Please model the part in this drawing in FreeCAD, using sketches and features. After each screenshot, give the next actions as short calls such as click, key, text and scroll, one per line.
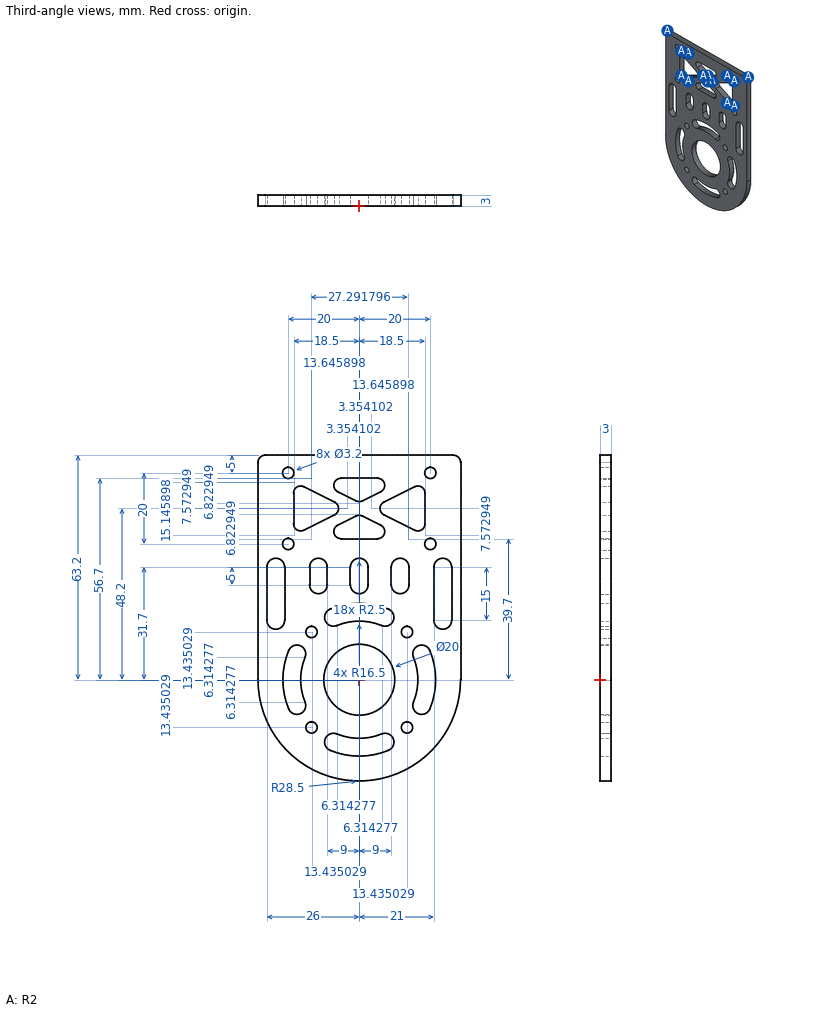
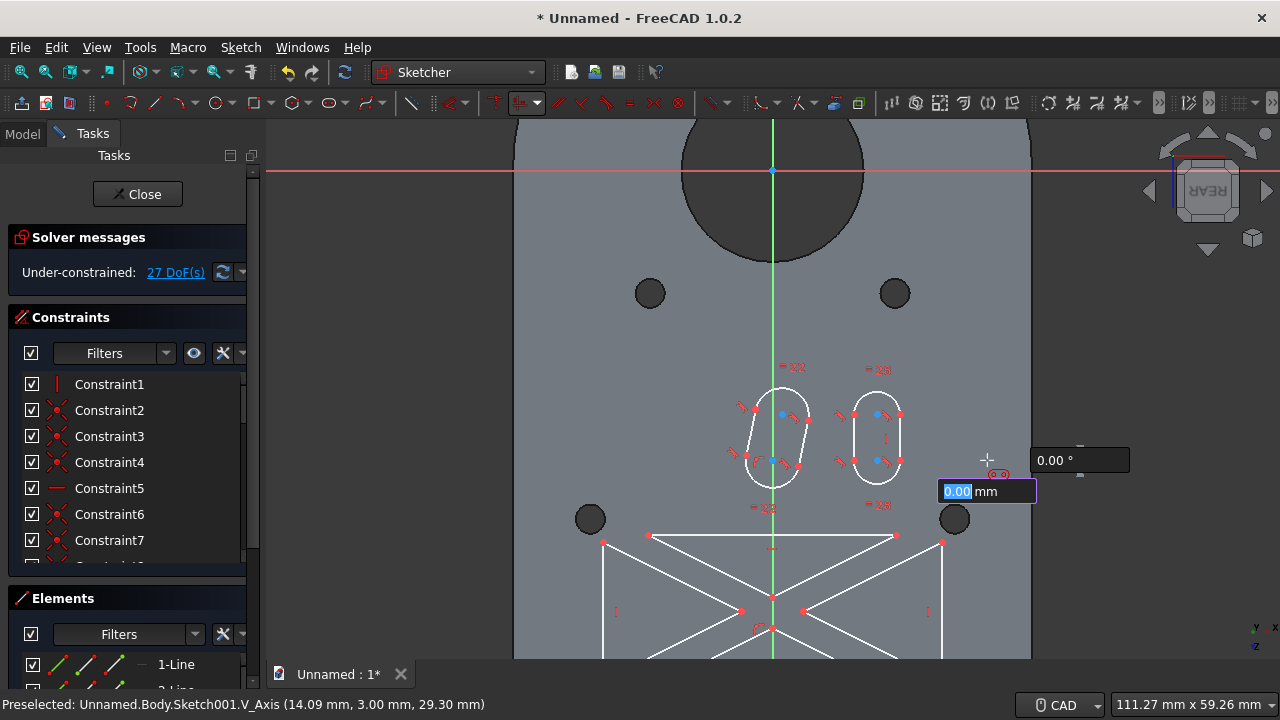
click(987, 323)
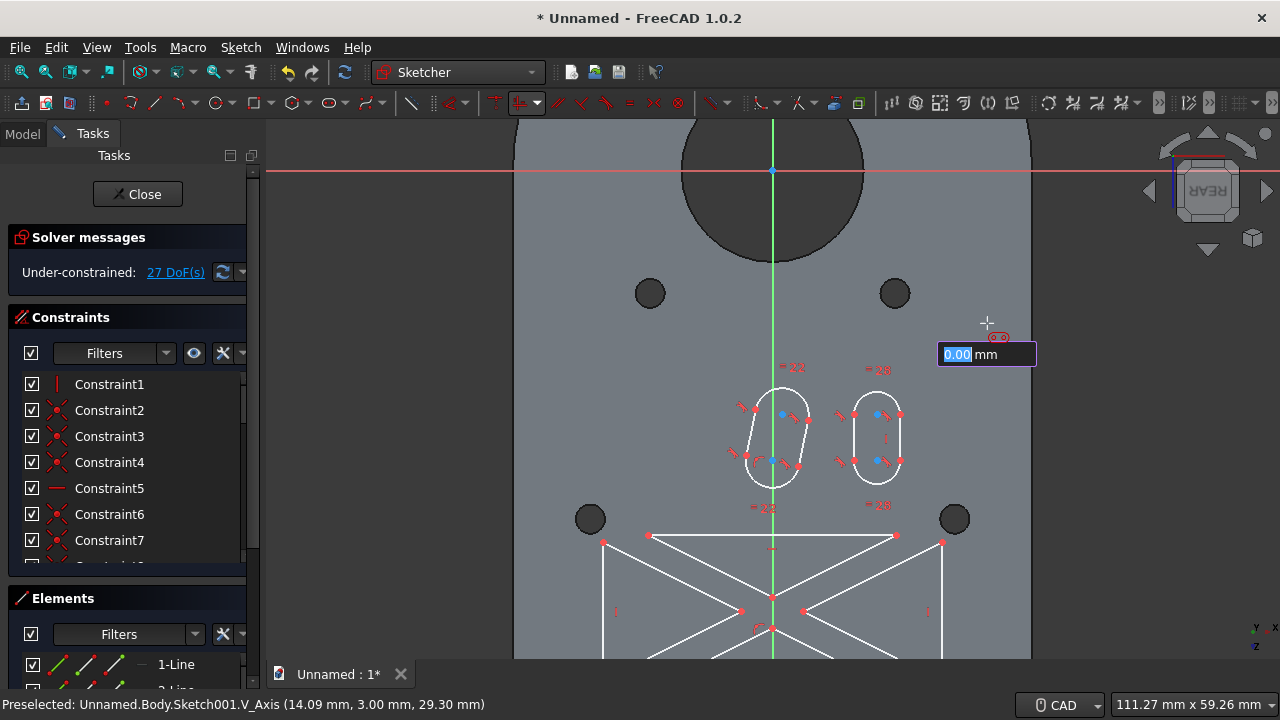
click(1010, 391)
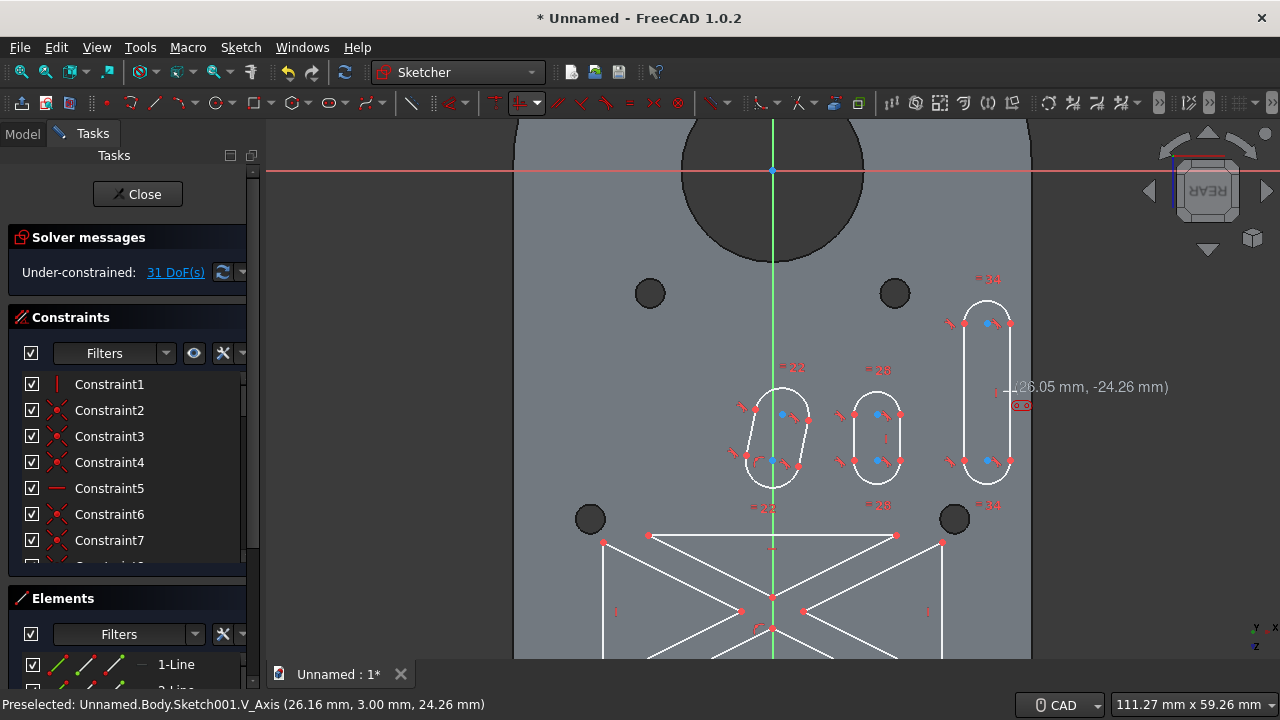
click(180, 104)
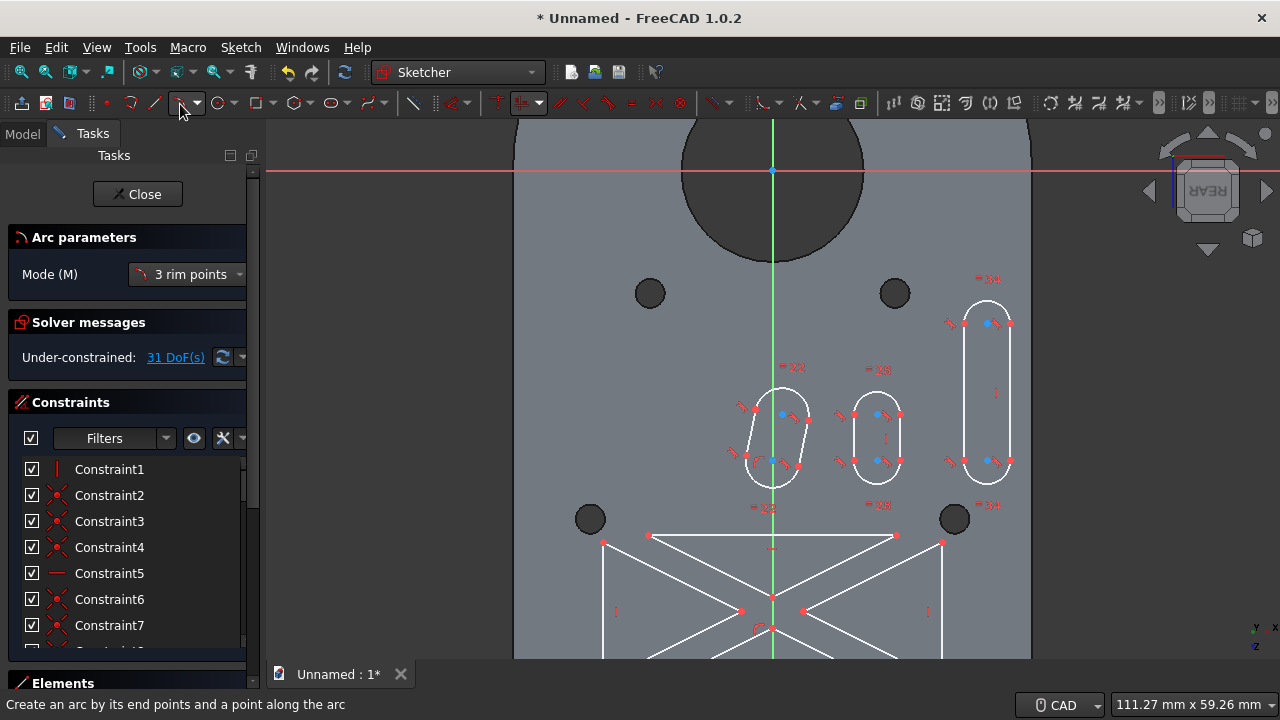
click(830, 310)
click(715, 310)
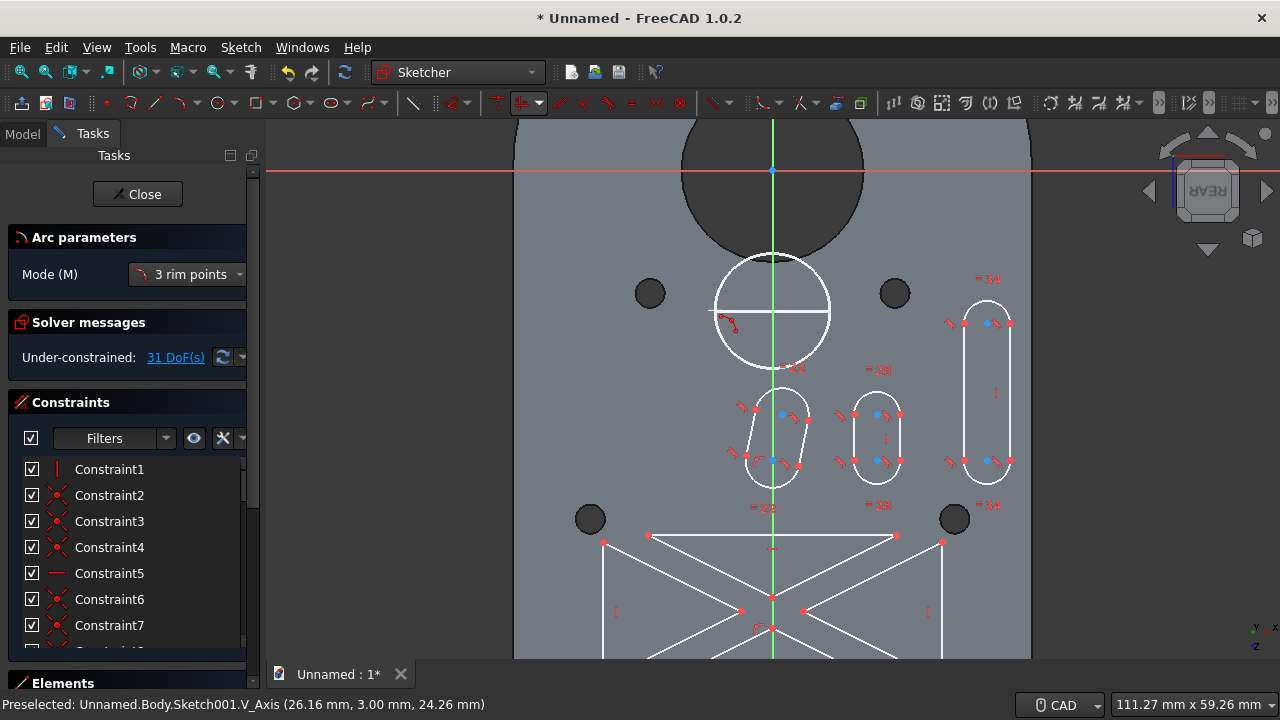
scroll(761, 321, up, 2)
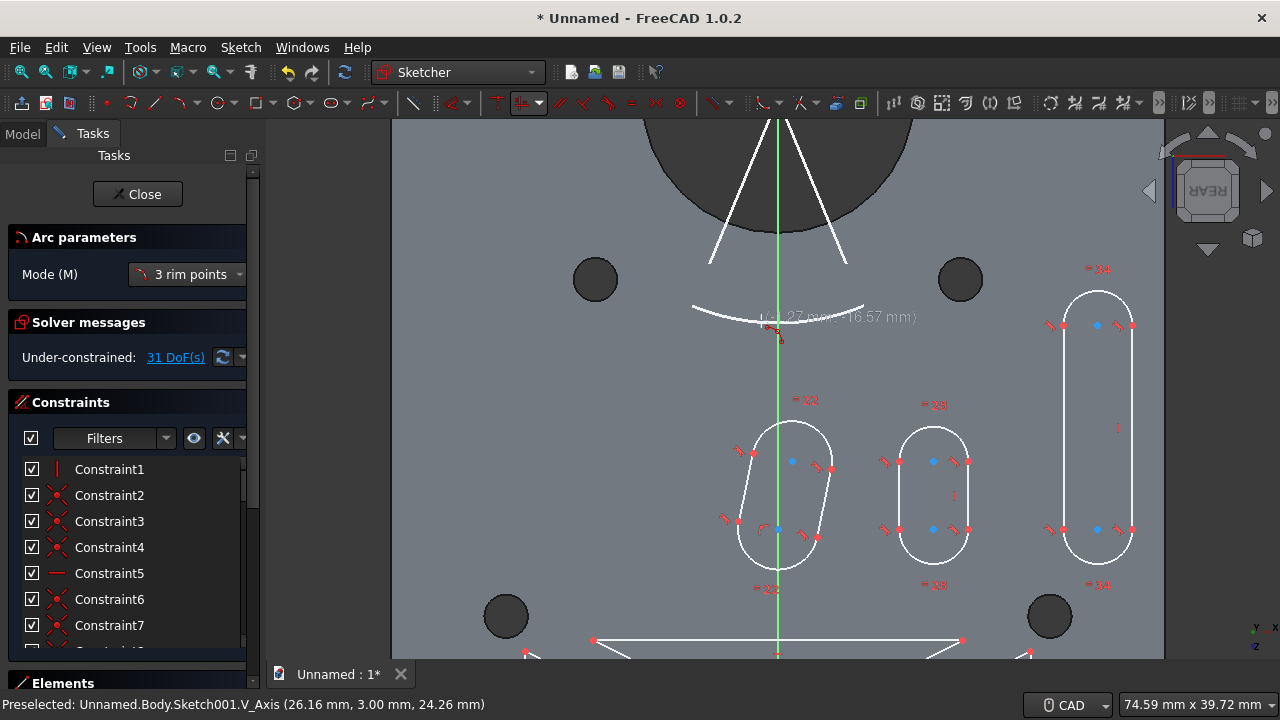
click(760, 321)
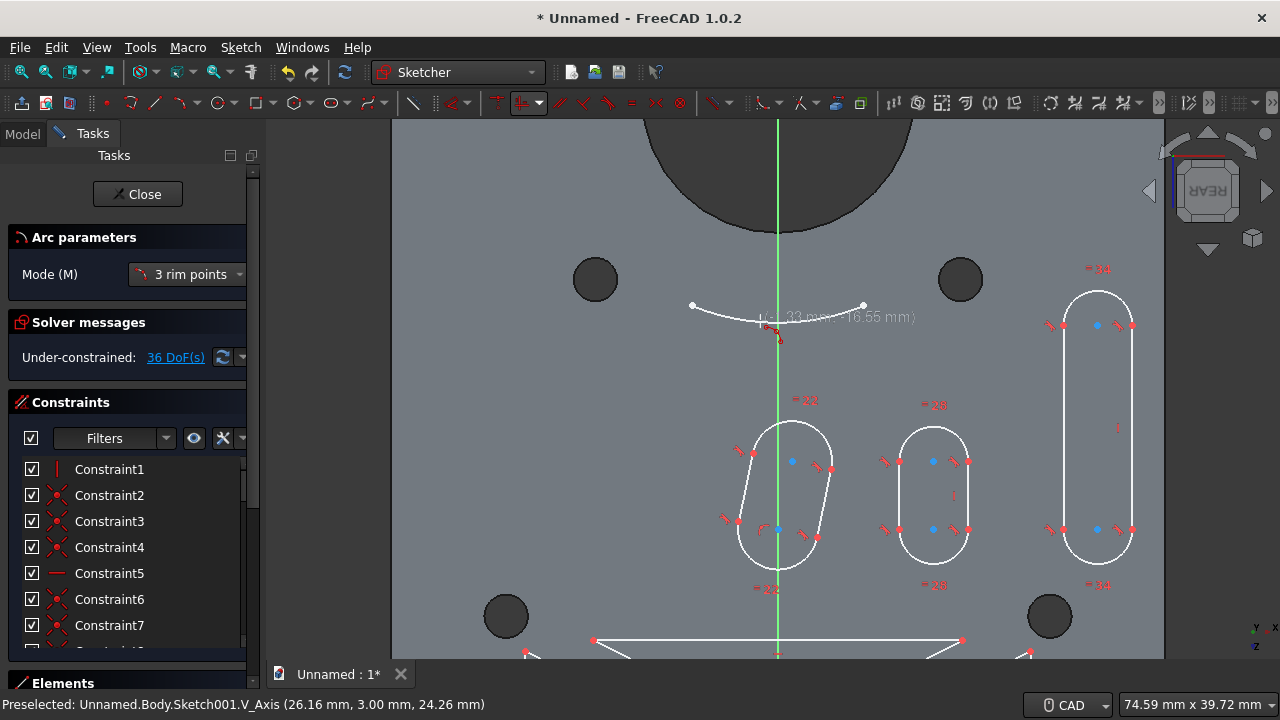
click(692, 306)
click(666, 367)
click(648, 323)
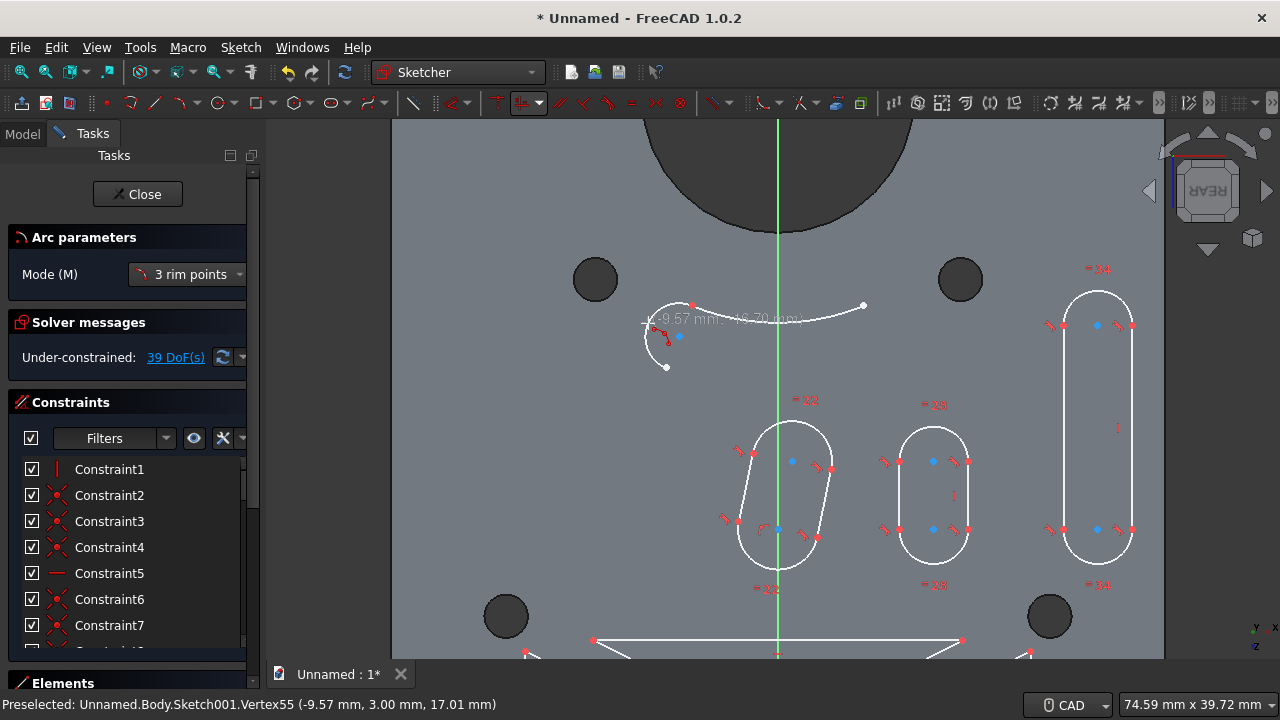
click(666, 368)
click(890, 367)
click(755, 388)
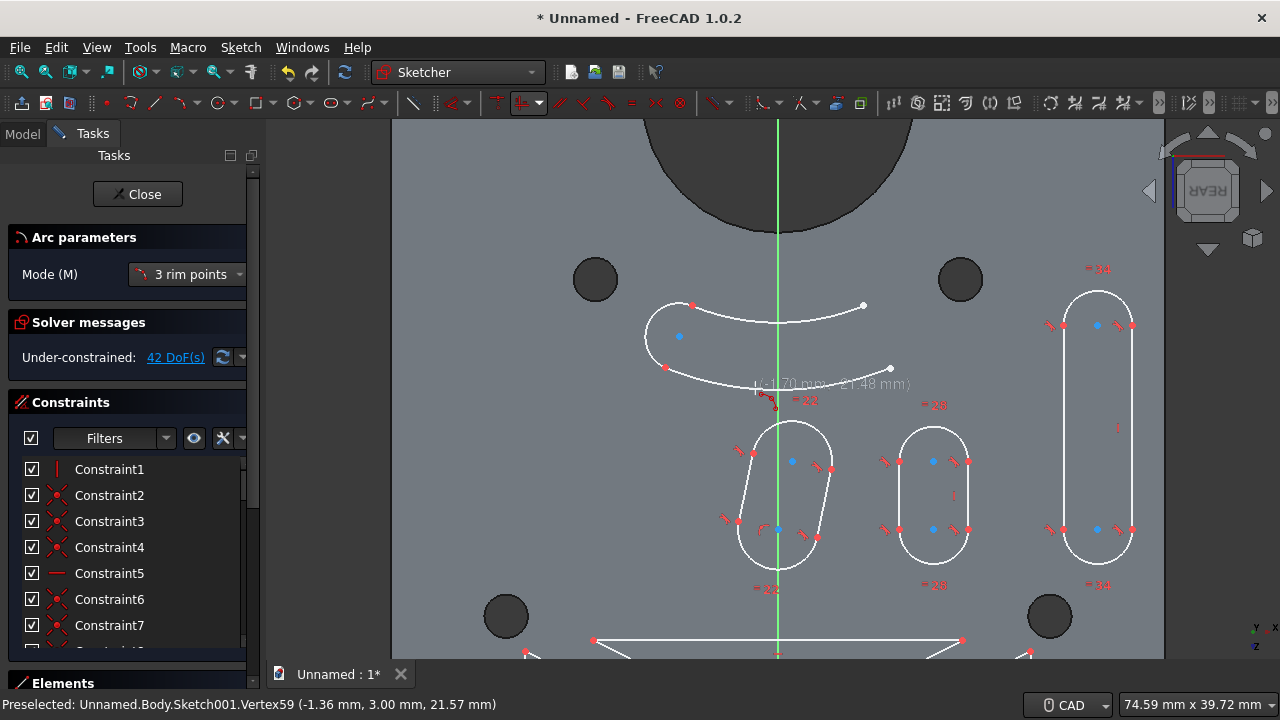
click(890, 368)
click(864, 306)
click(908, 323)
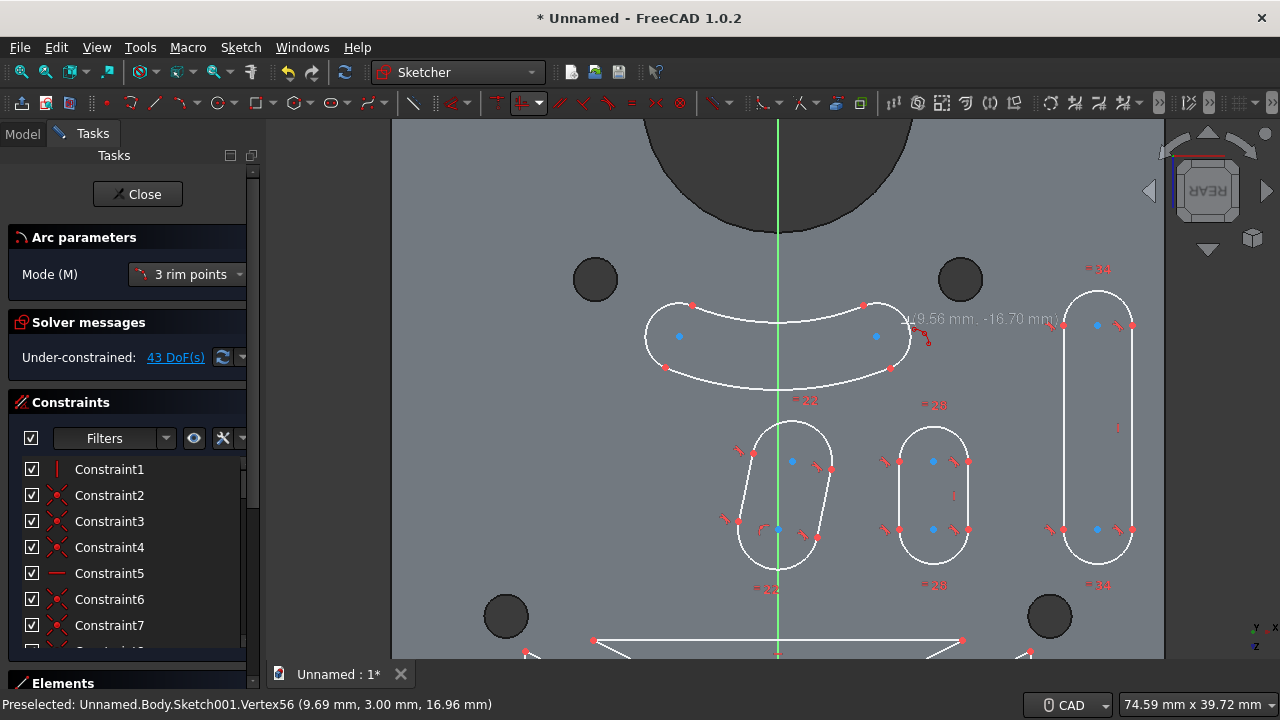
key(g)
key(s)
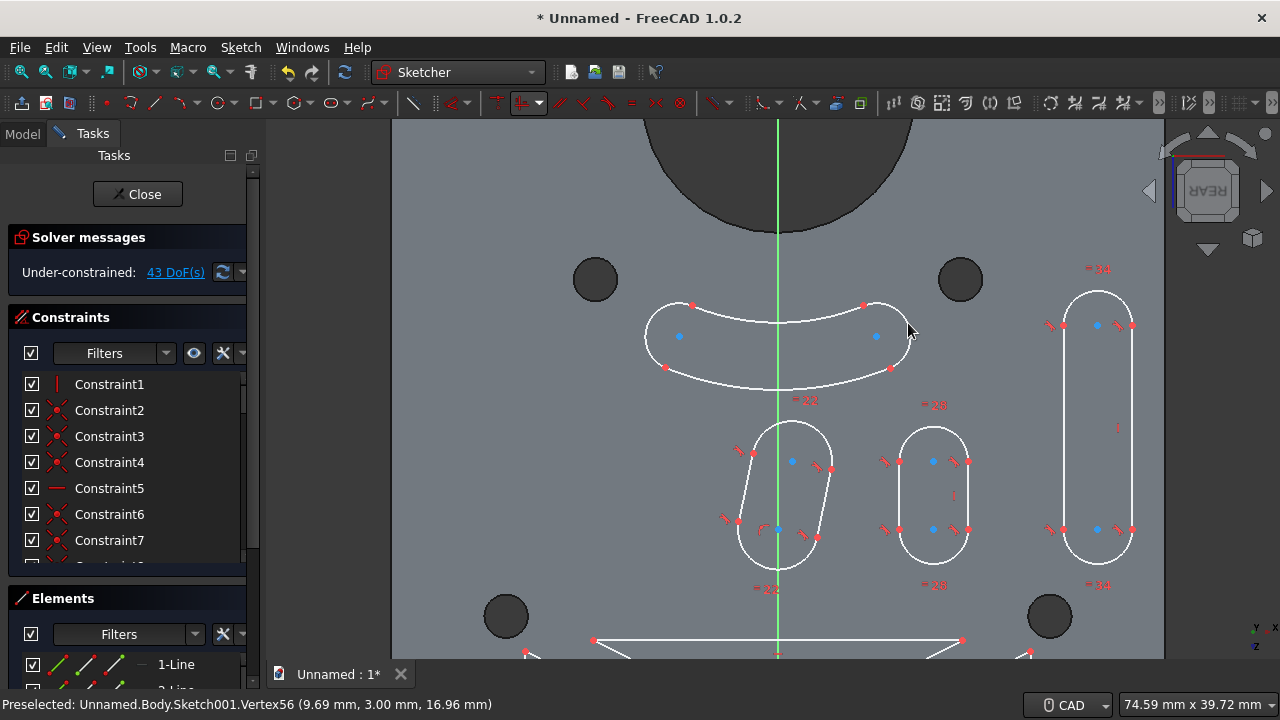
click(622, 528)